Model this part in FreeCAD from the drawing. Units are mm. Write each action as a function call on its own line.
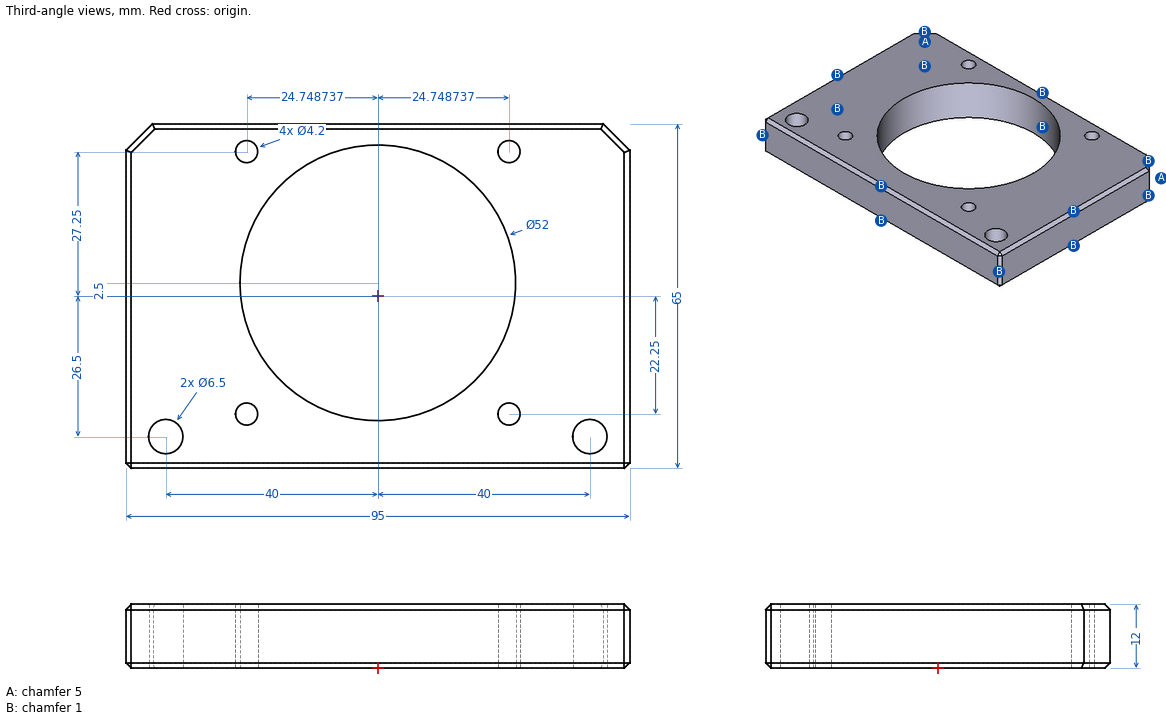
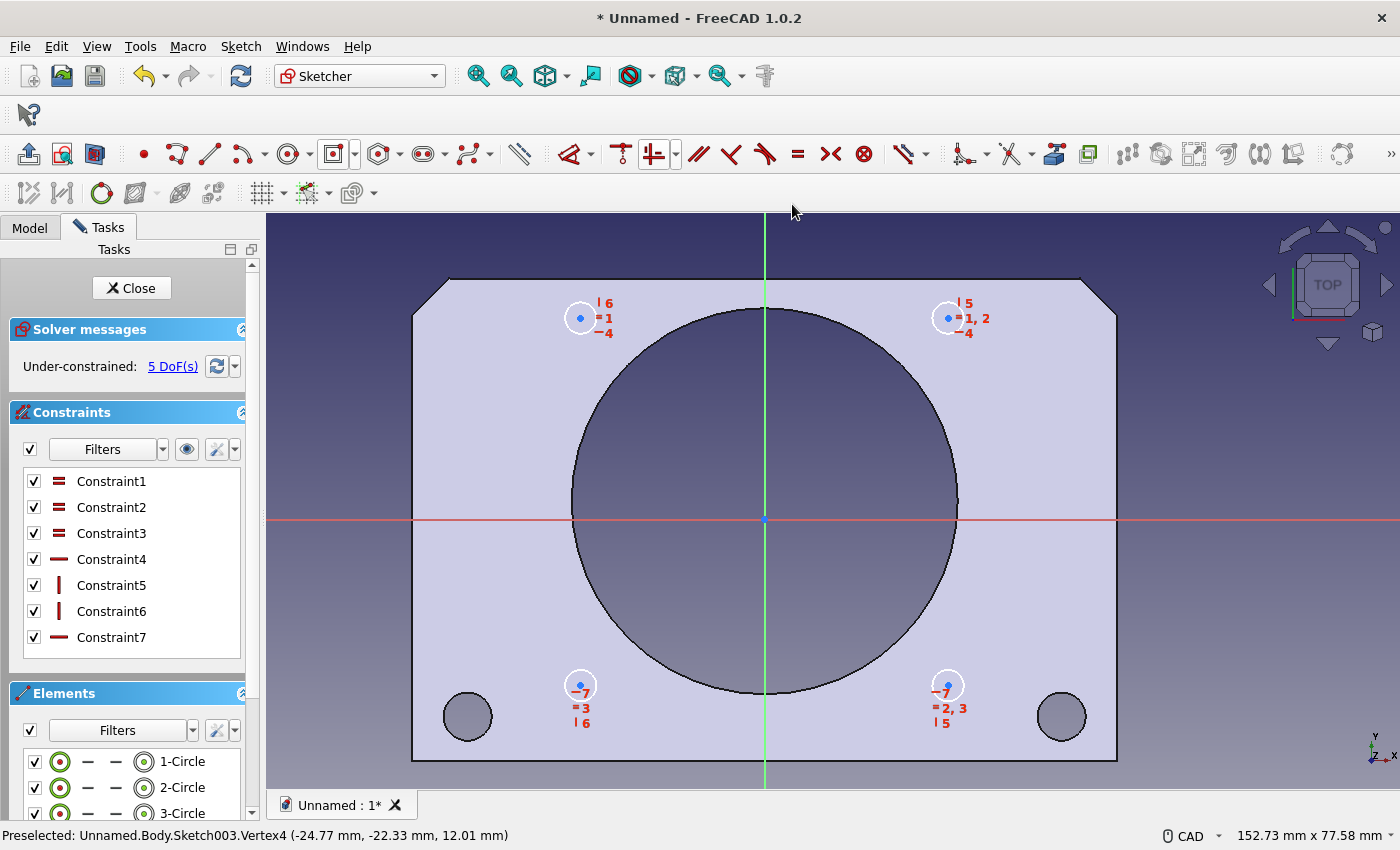
scroll(592, 307, up, 2)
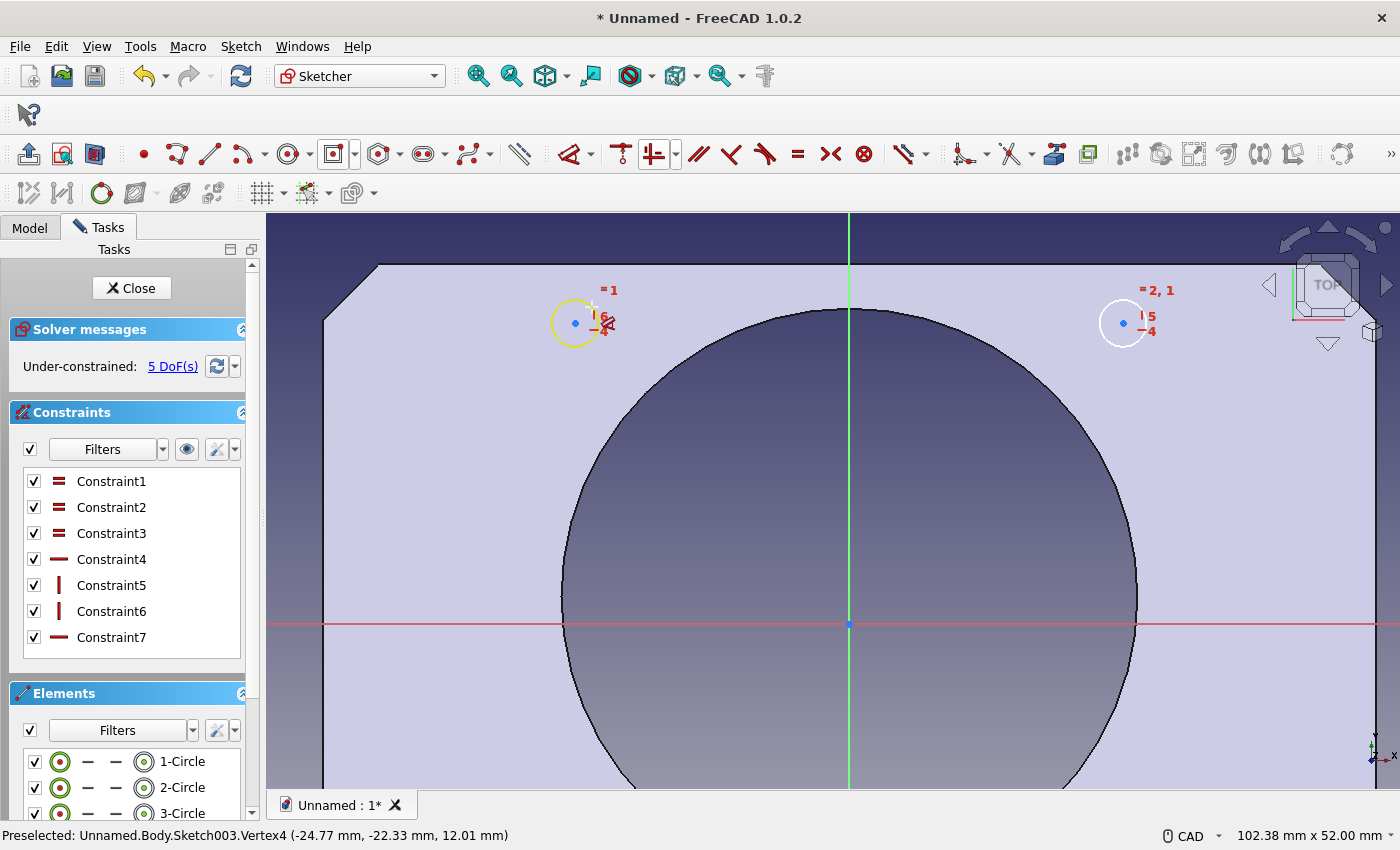
click(592, 307)
click(615, 285)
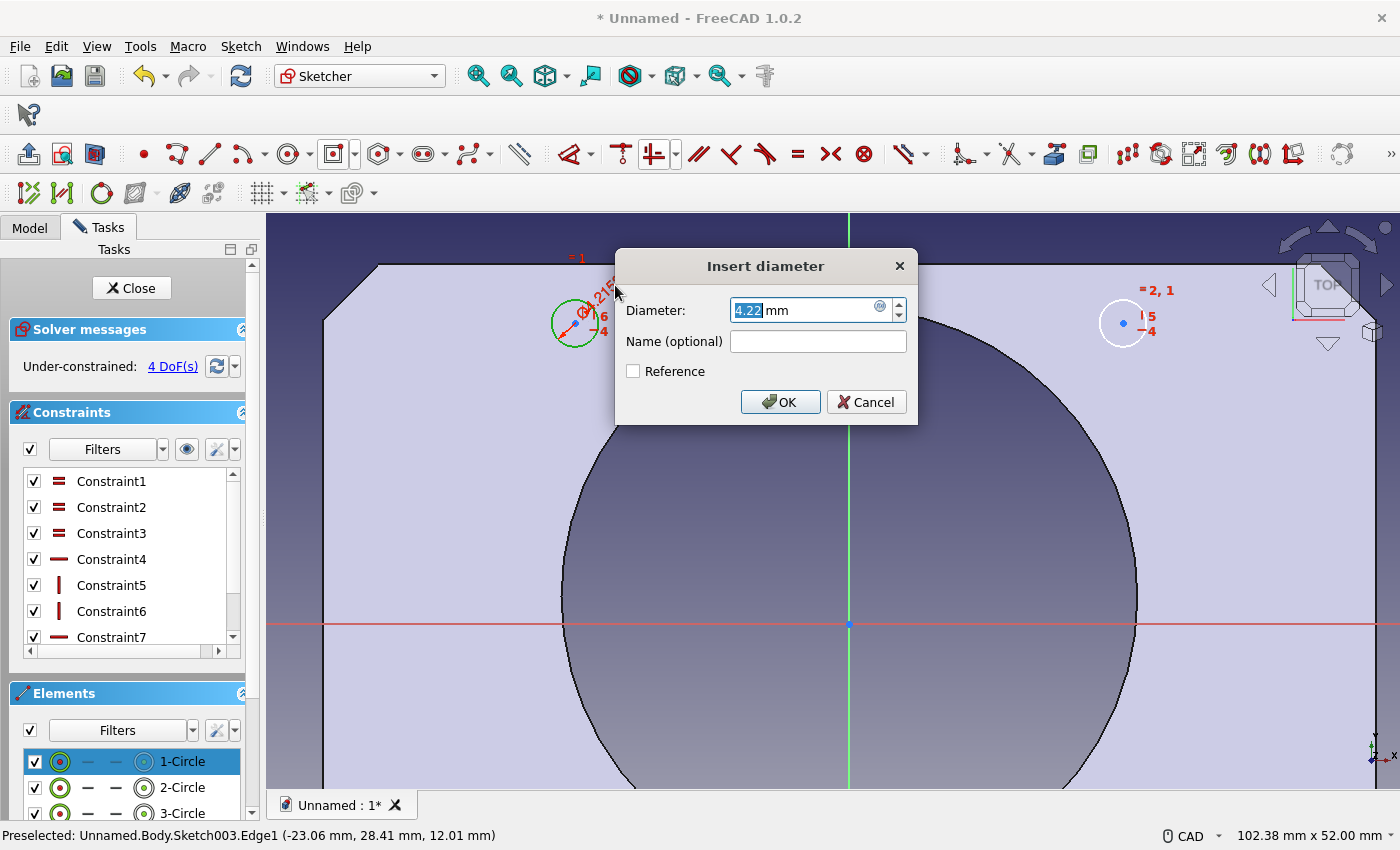
text(4.2)
key(Return)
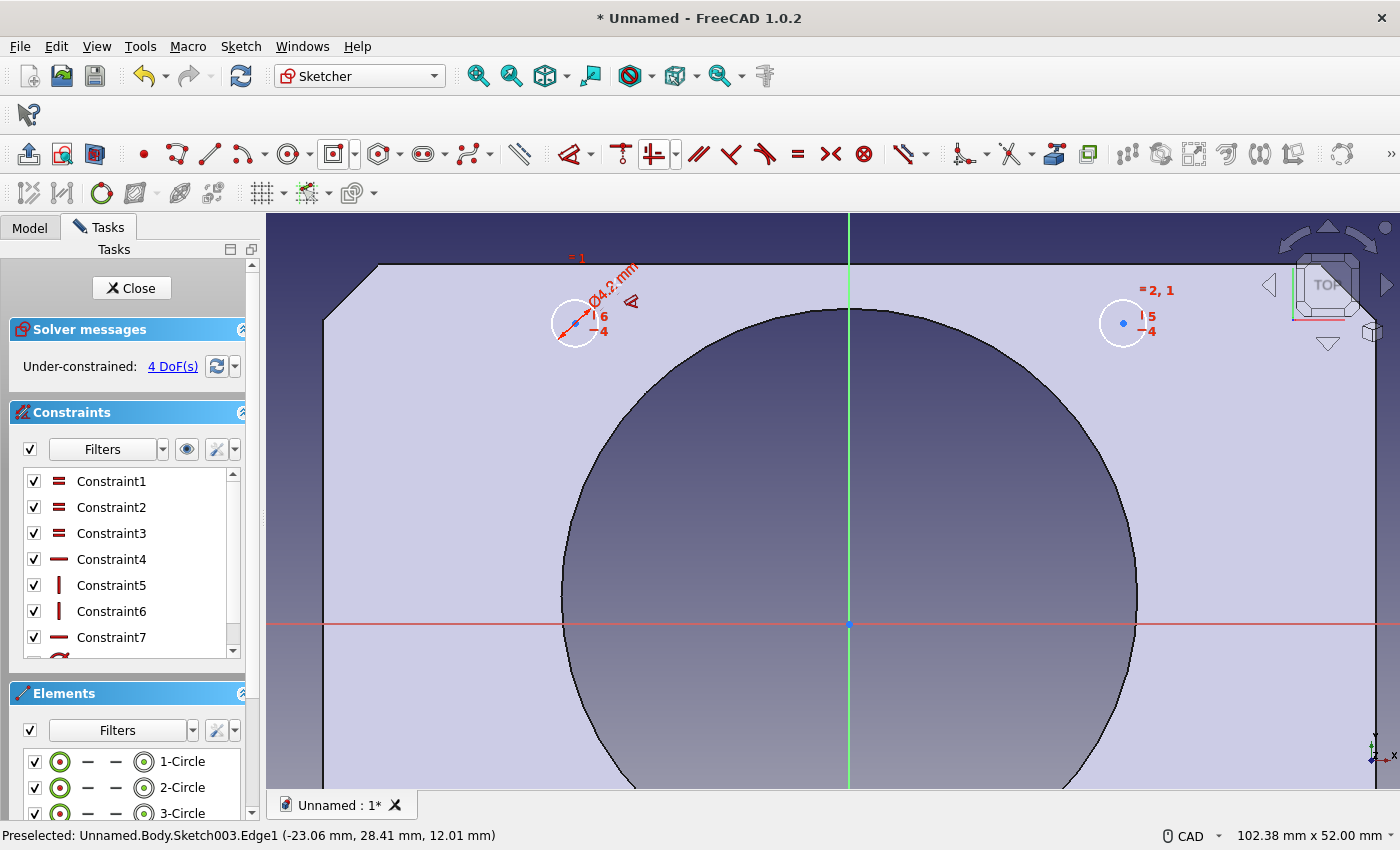
click(575, 323)
click(541, 474)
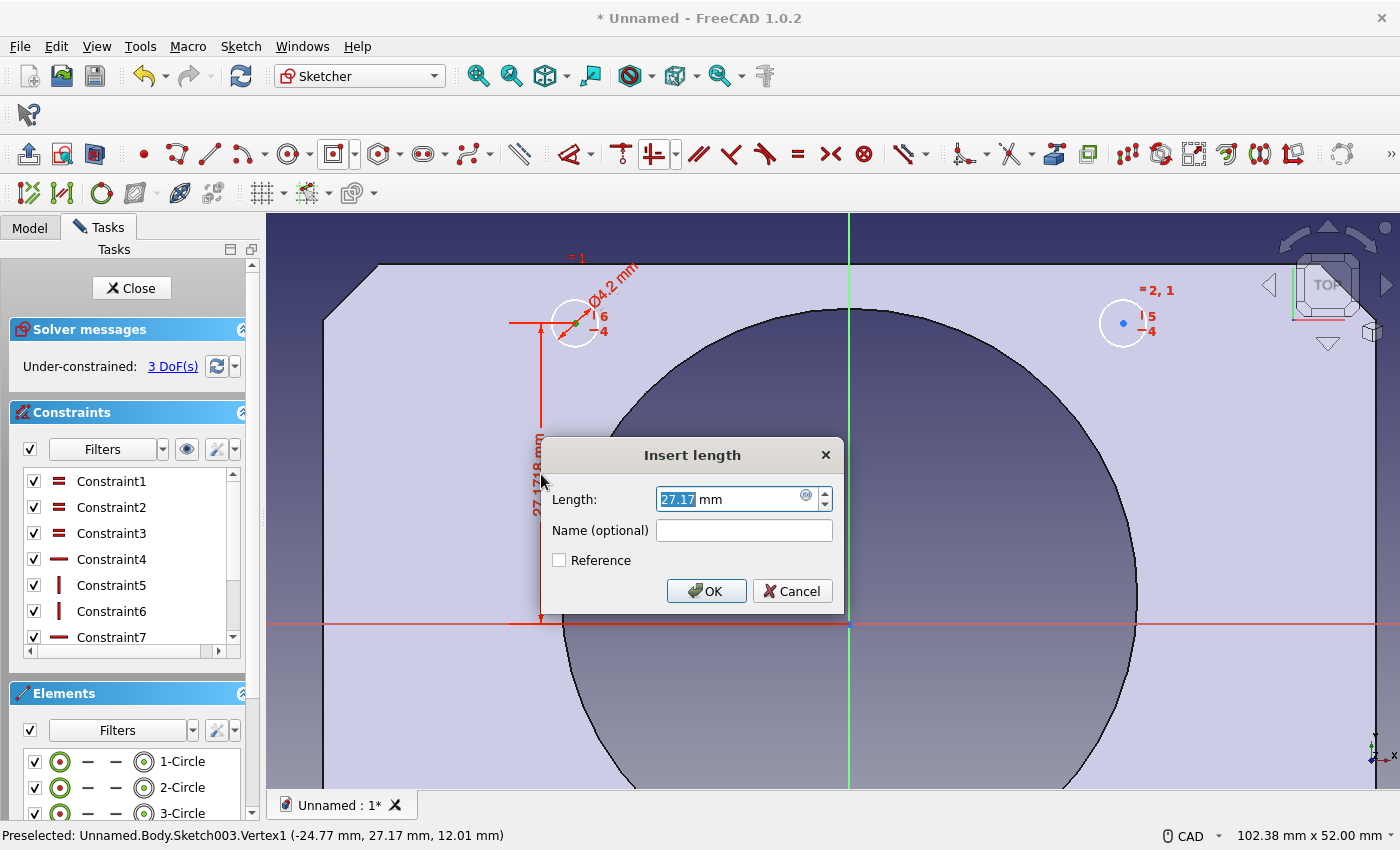
text(27.25)
key(Return)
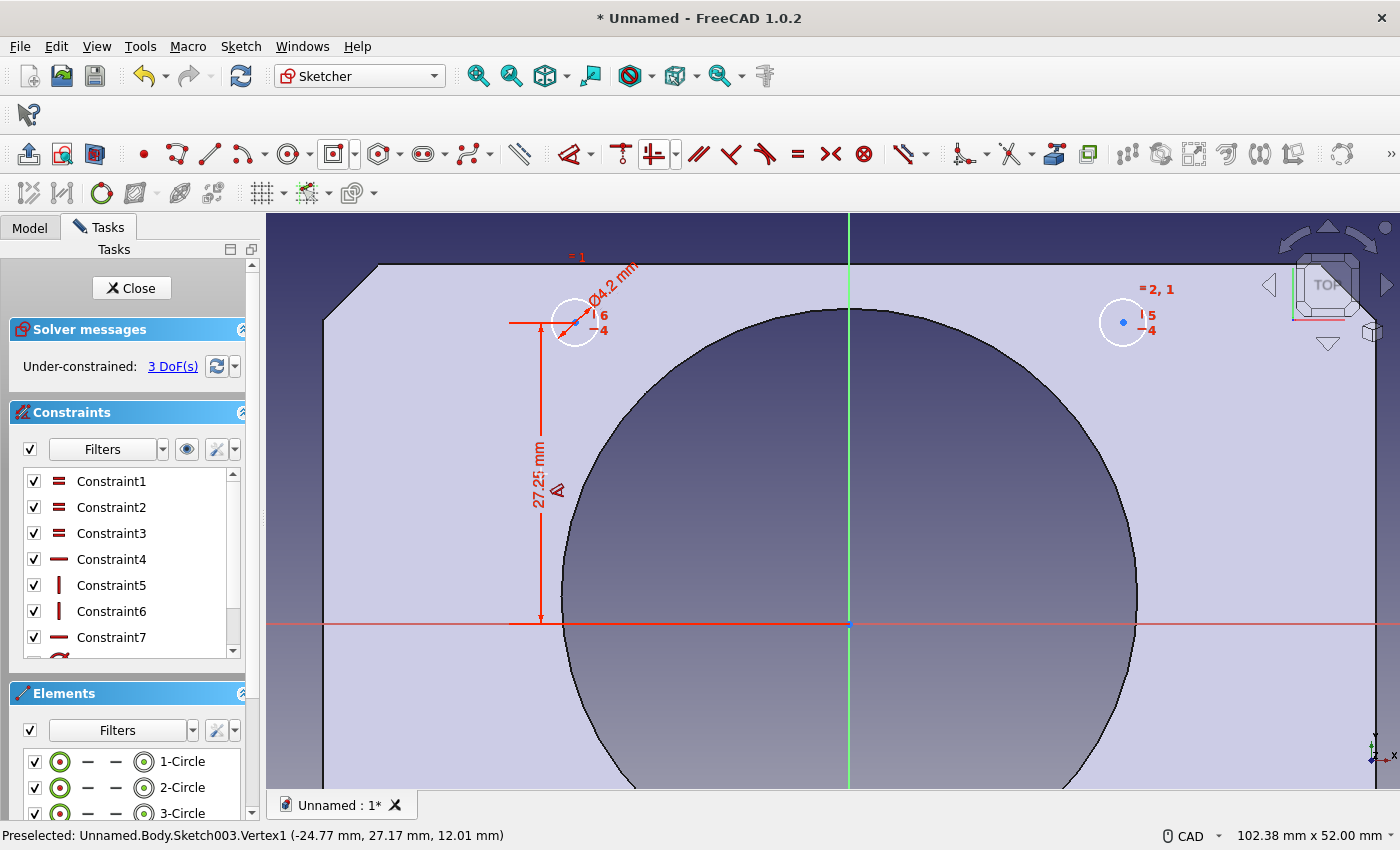
scroll(592, 306, down, 2)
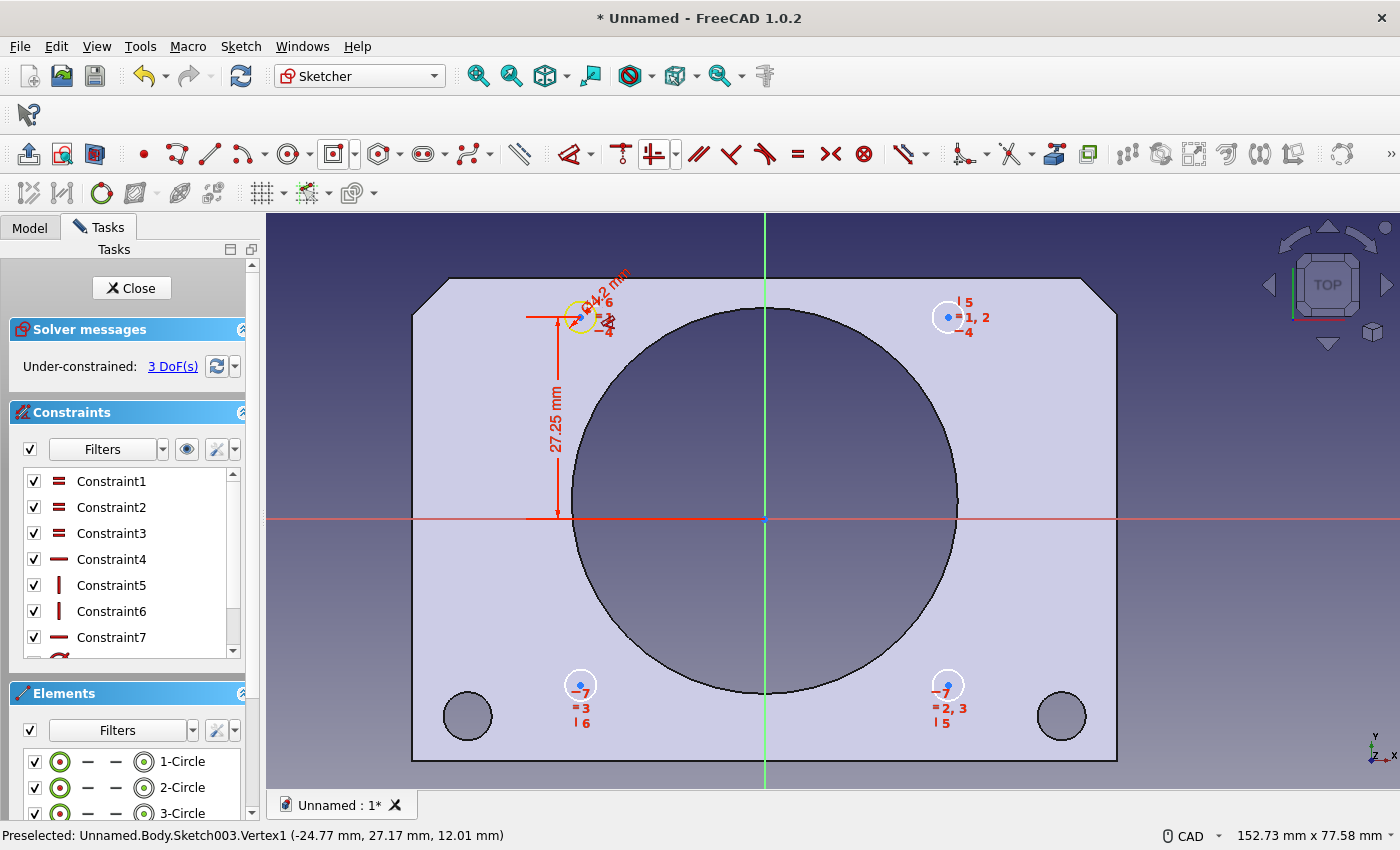
click(948, 685)
click(982, 602)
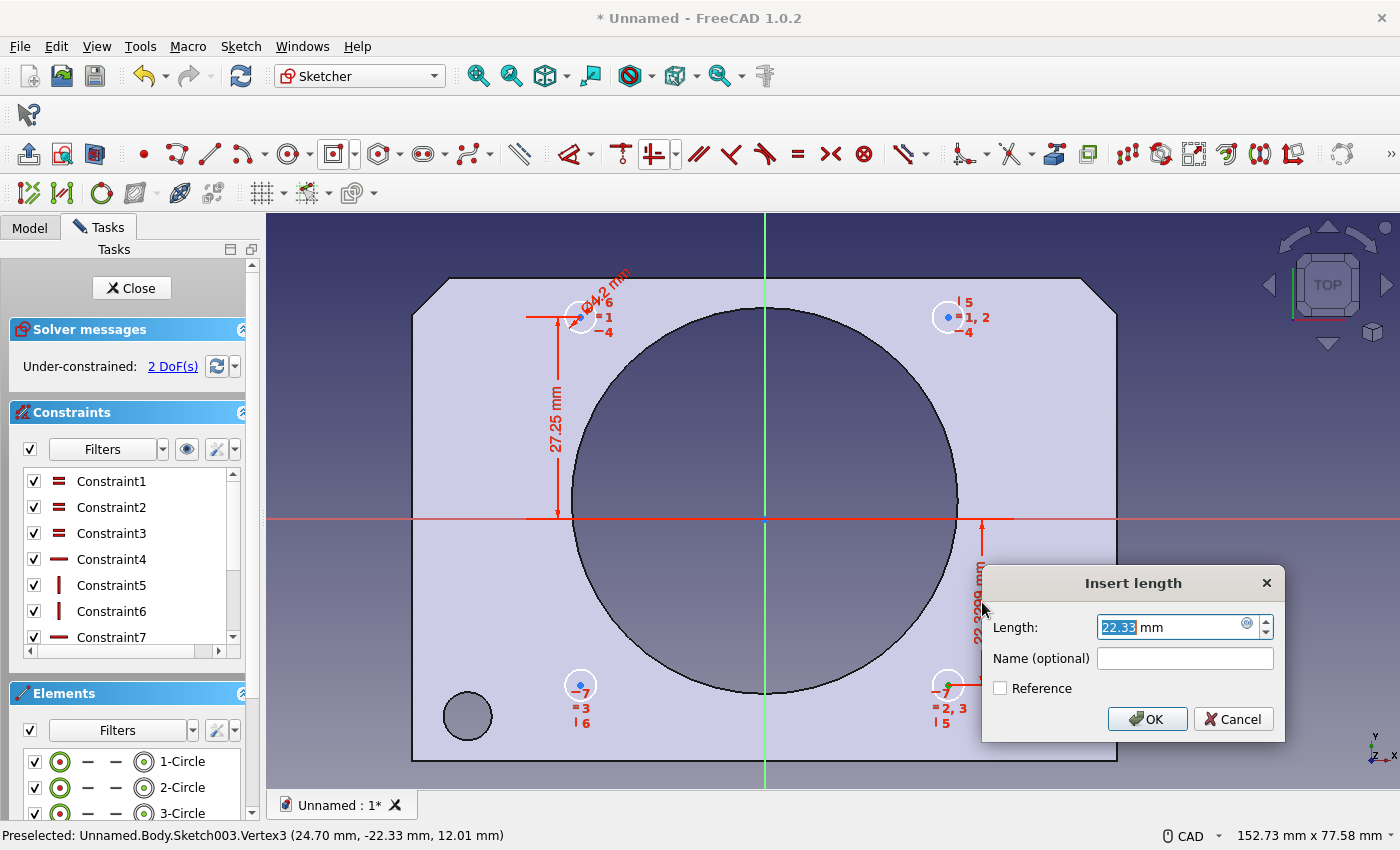
text(22.25)
key(Return)